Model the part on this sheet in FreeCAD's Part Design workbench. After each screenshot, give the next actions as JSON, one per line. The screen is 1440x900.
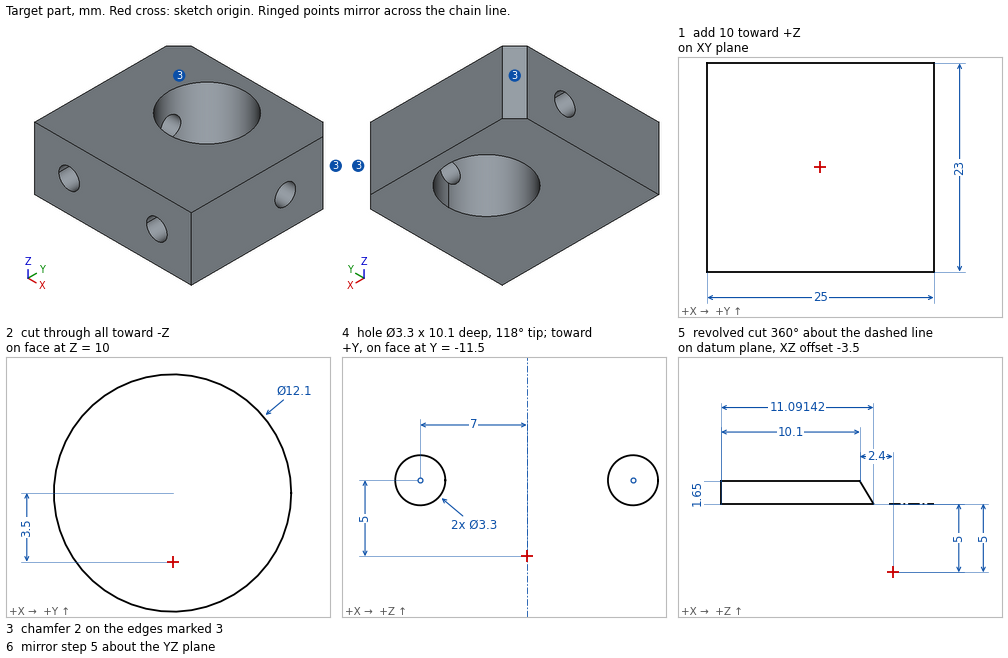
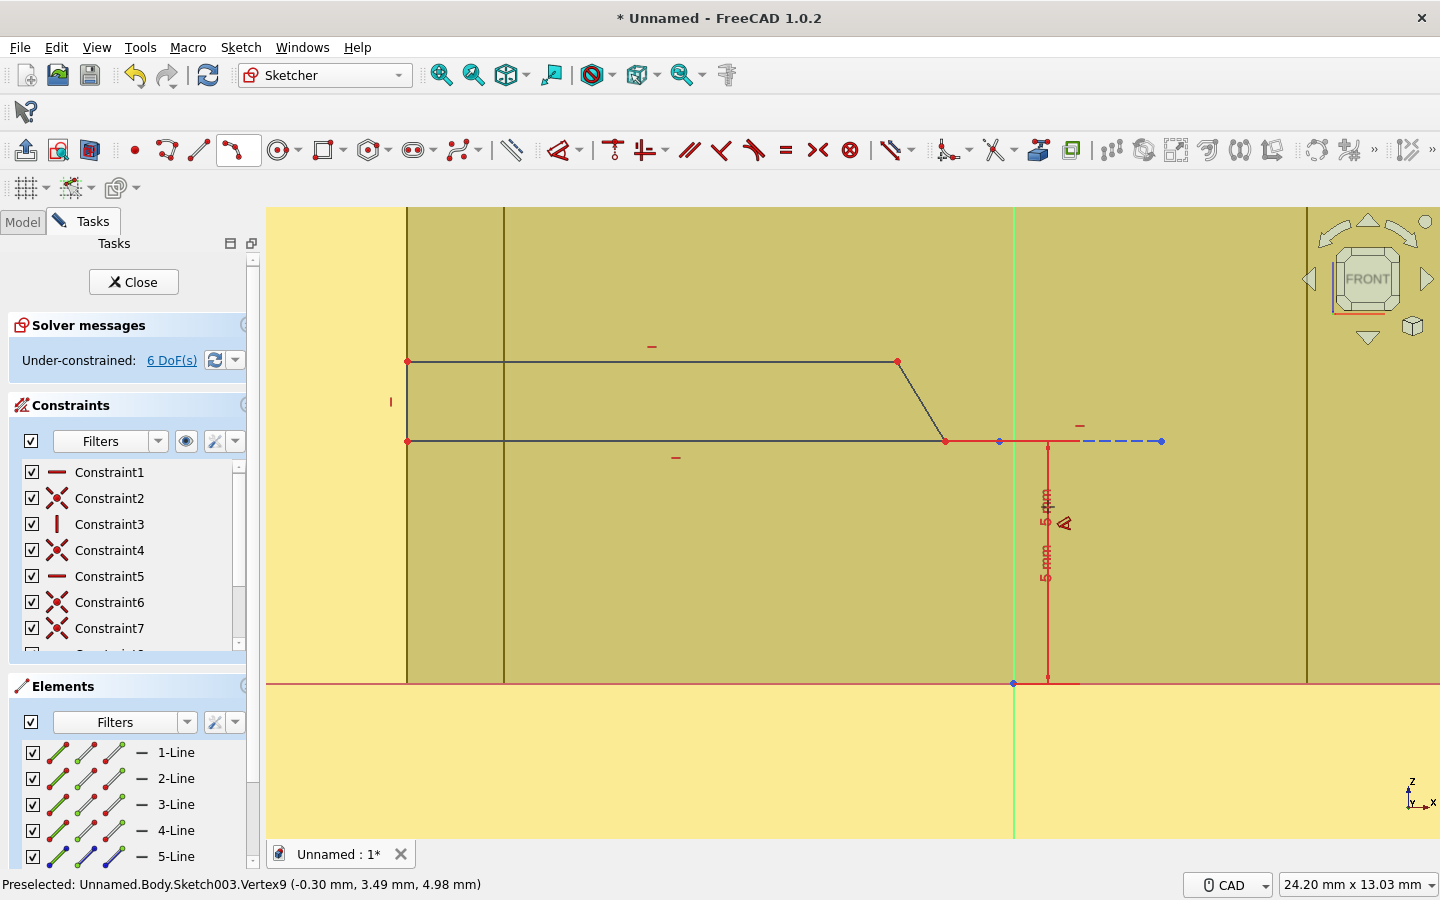
{"action": "left_click", "coordinate": [407, 417]}
{"action": "left_click", "coordinate": [373, 402]}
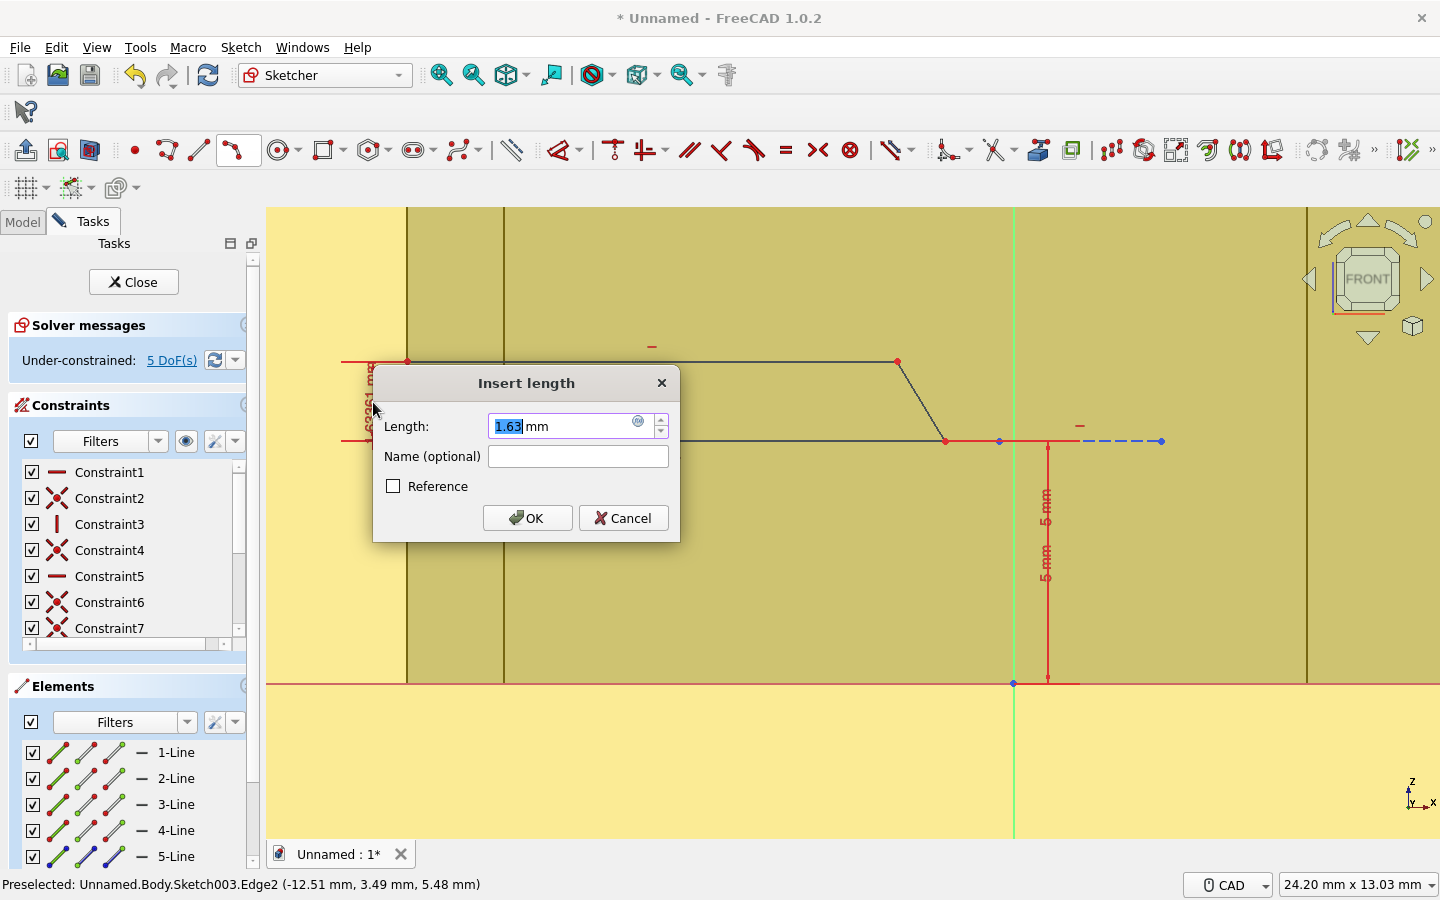
{"action": "type", "text": "1.65"}
{"action": "key", "text": "Return"}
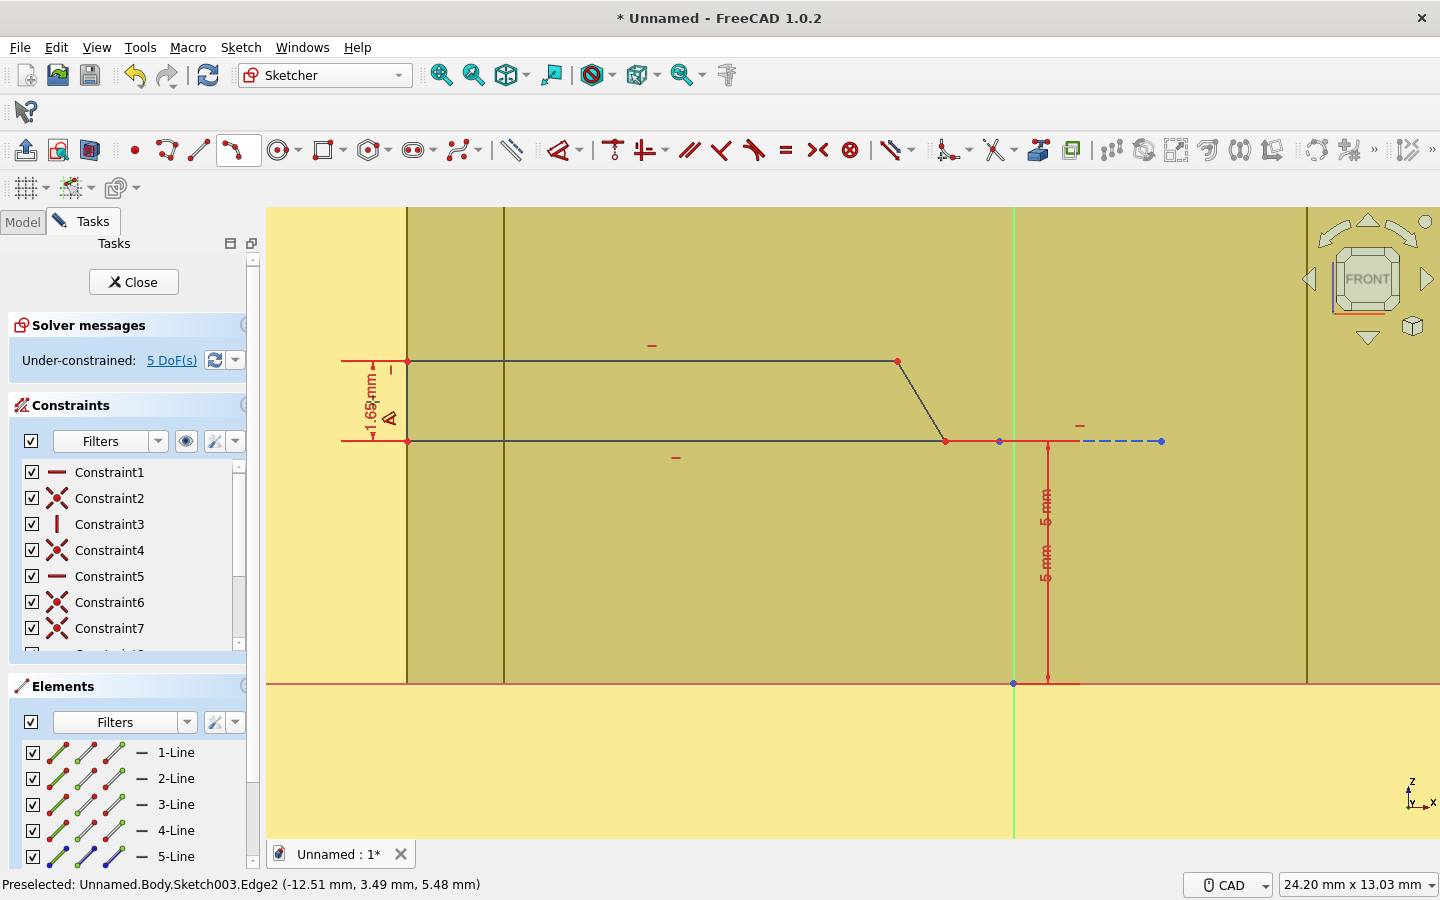
{"action": "left_click", "coordinate": [554, 361]}
{"action": "left_click", "coordinate": [652, 327]}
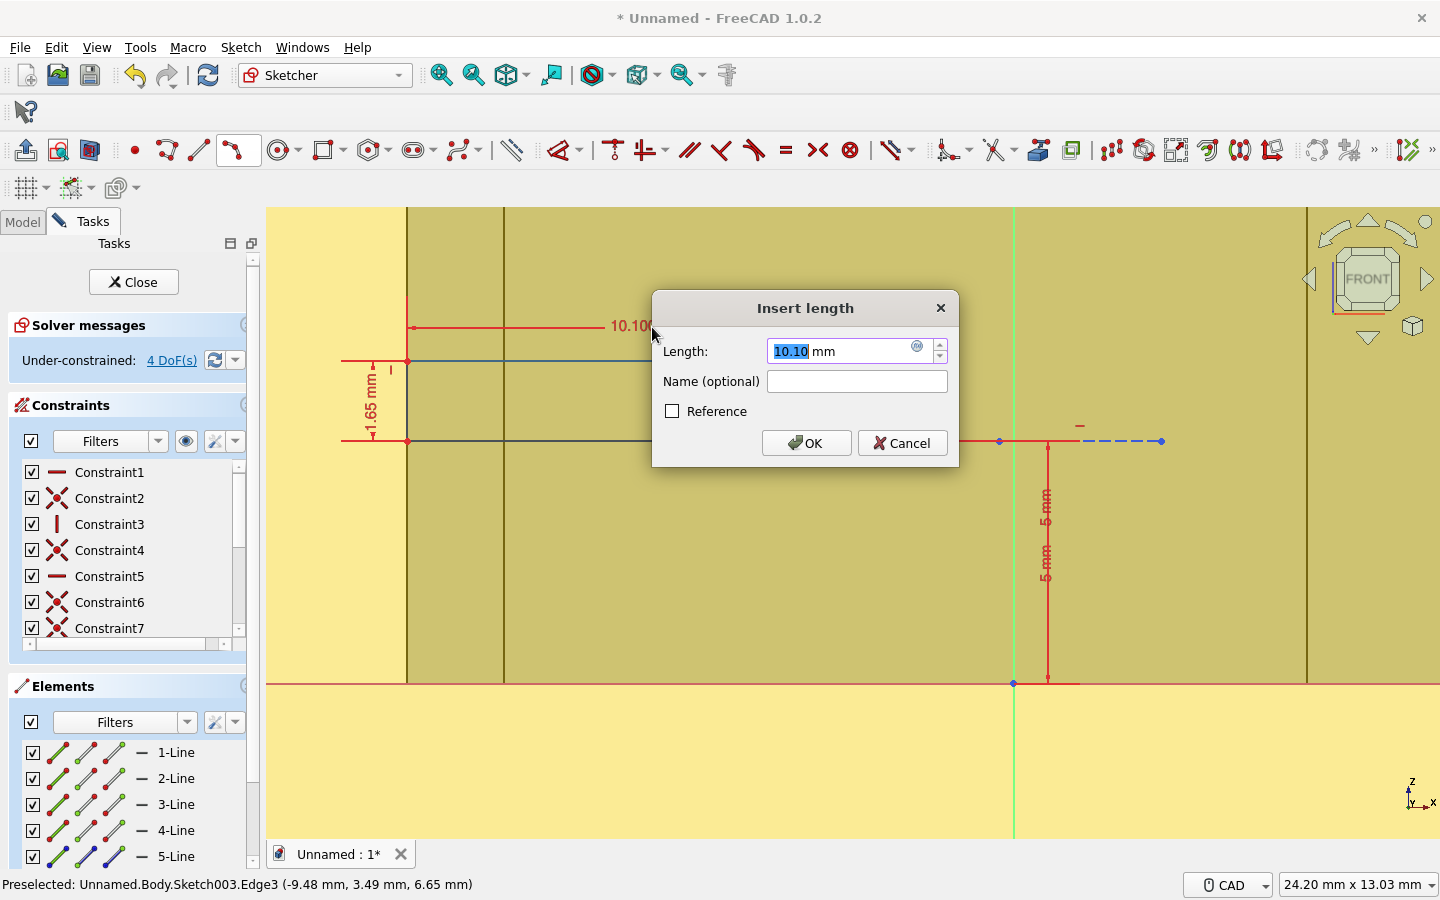
{"action": "type", "text": "10.1"}
{"action": "key", "text": "Return"}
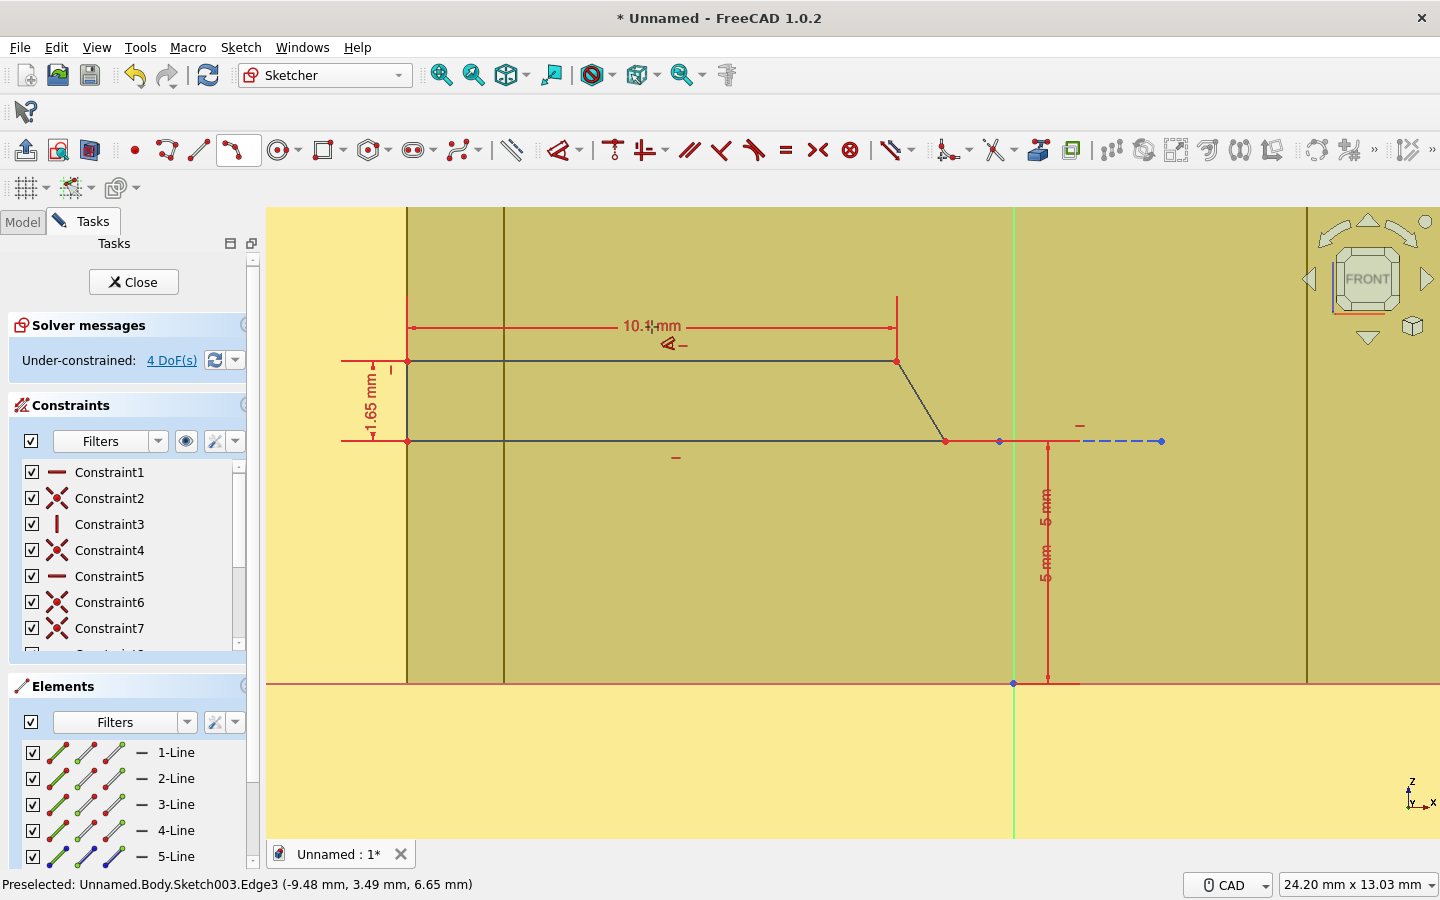
{"action": "left_click", "coordinate": [897, 361]}
{"action": "left_click", "coordinate": [955, 718]}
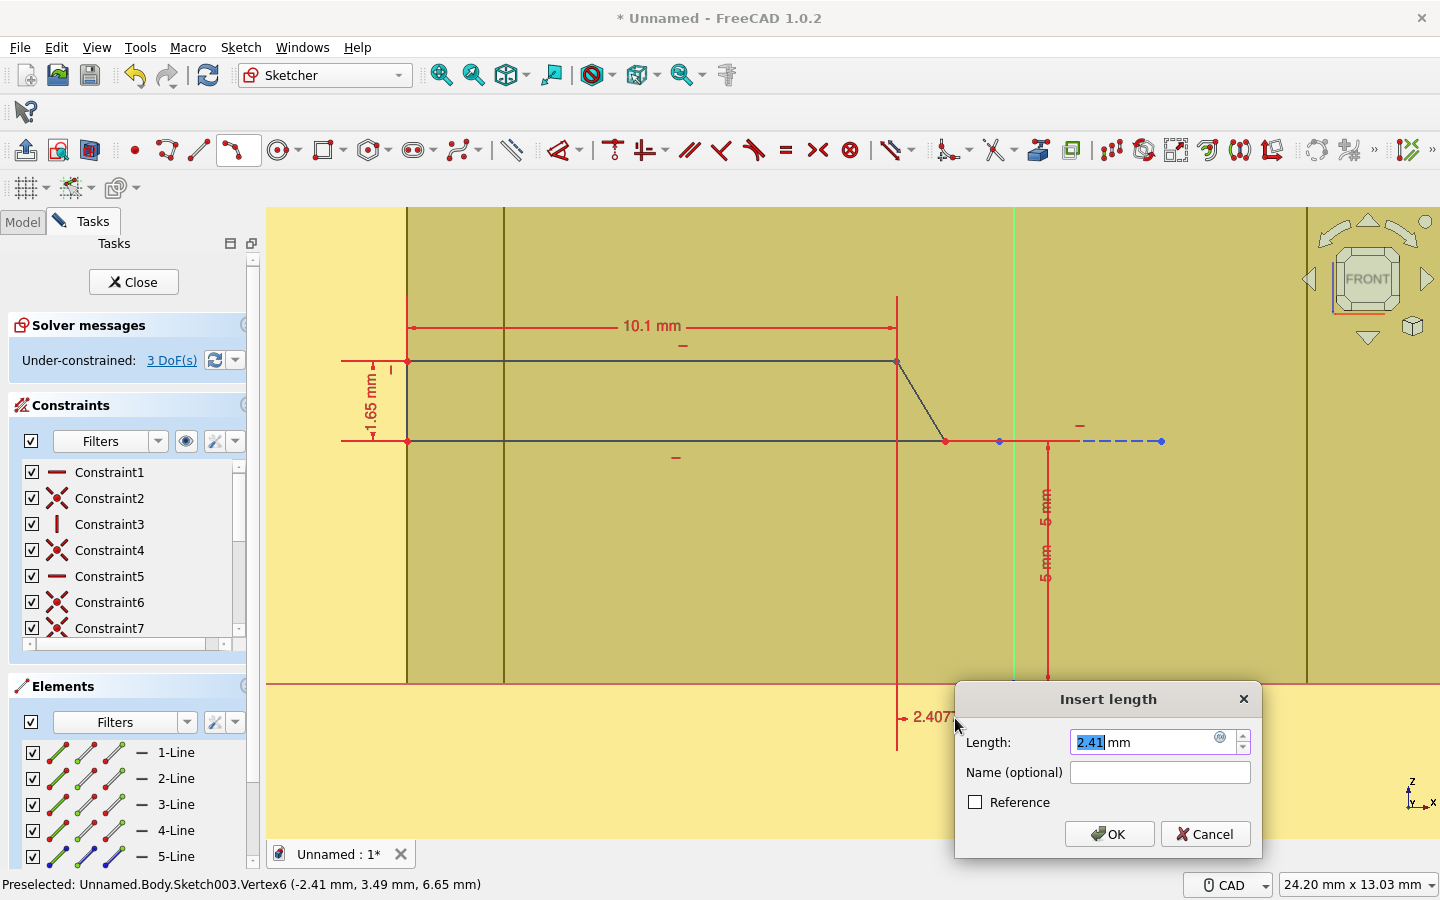
{"action": "type", "text": "2.4"}
{"action": "key", "text": "Return"}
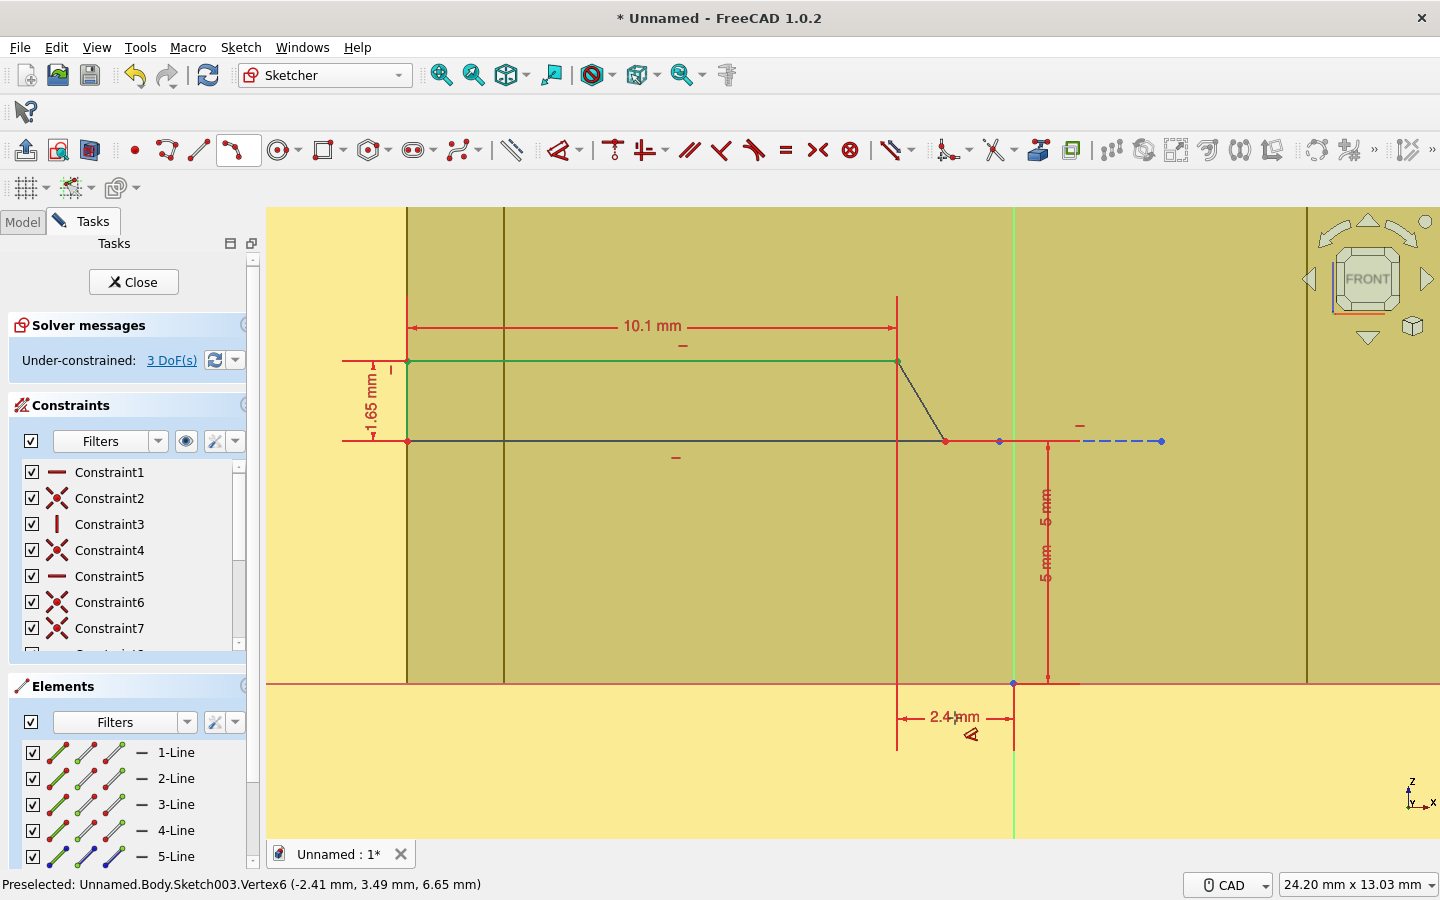
{"action": "left_click", "coordinate": [784, 441]}
{"action": "left_click", "coordinate": [676, 407]}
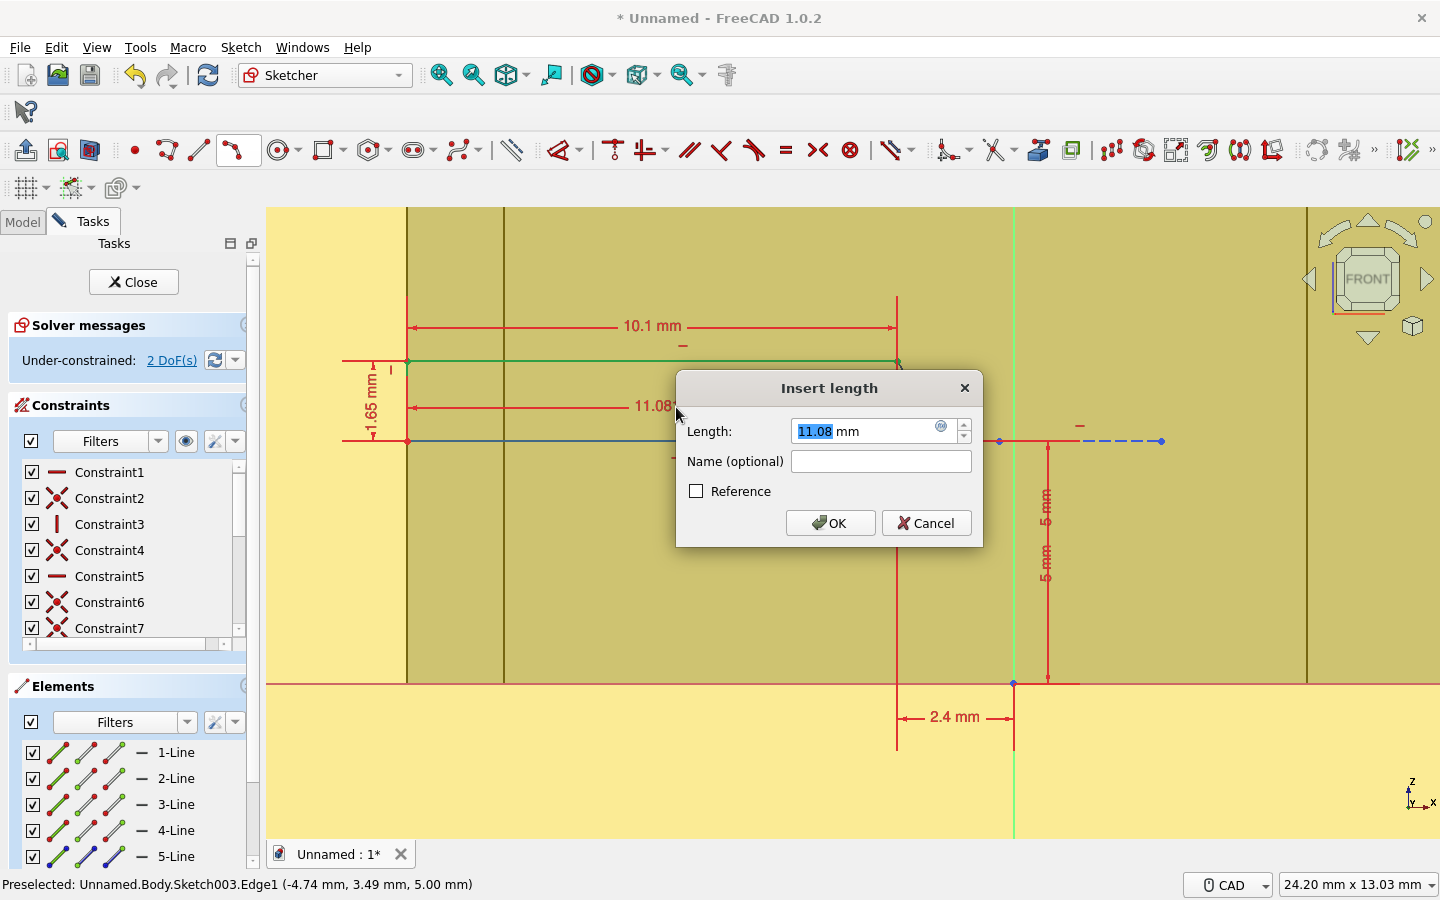
{"action": "type", "text": "11.09142"}
{"action": "key", "text": "Return"}
{"action": "key", "text": "Escape"}